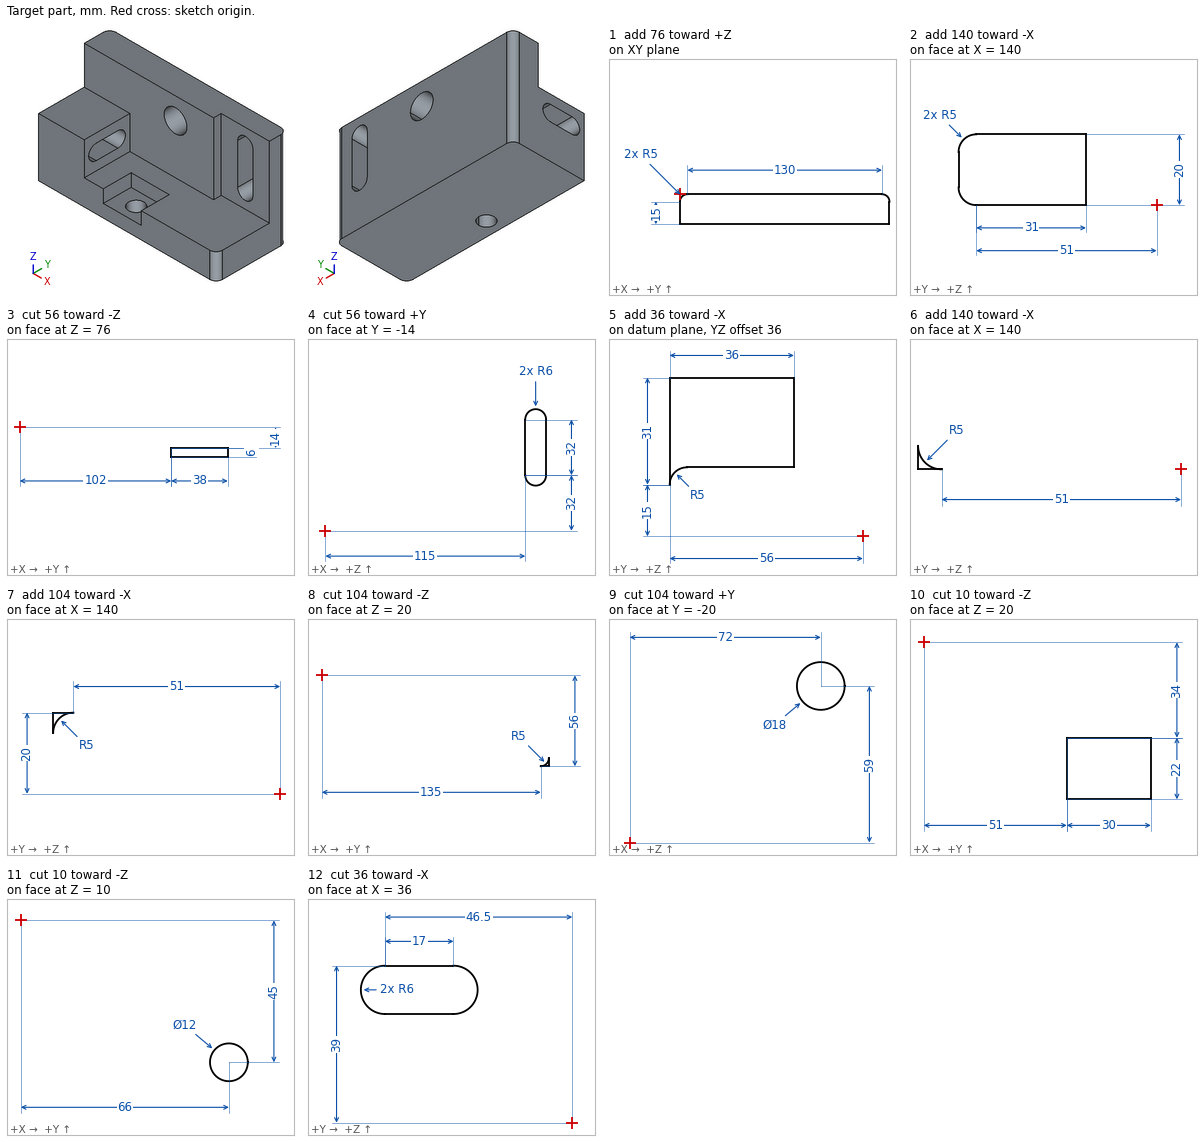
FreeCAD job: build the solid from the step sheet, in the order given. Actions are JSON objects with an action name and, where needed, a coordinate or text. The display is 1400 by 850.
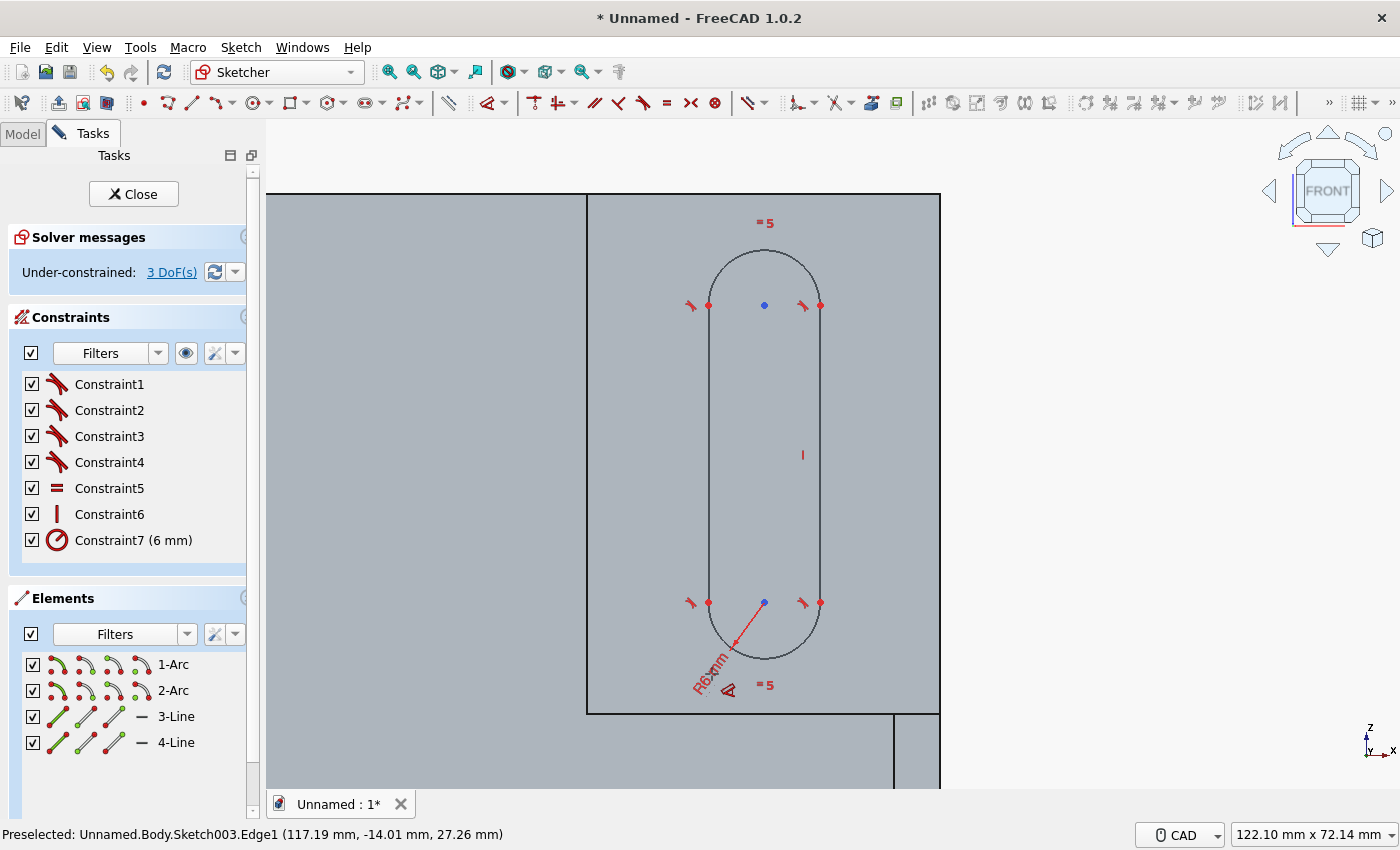
{"action": "left_click", "coordinate": [709, 514]}
{"action": "left_click", "coordinate": [675, 455]}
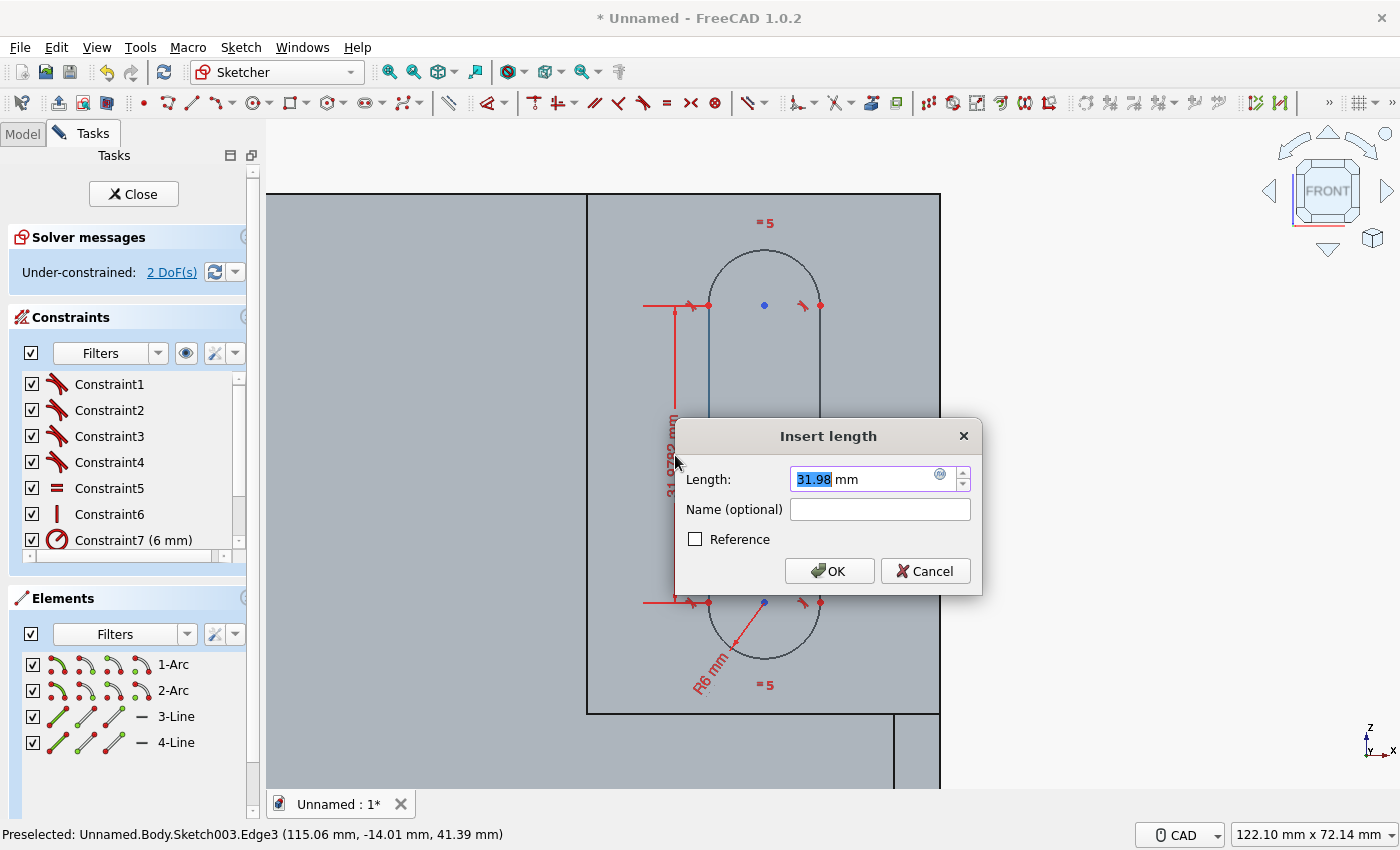
{"action": "type", "text": "32"}
{"action": "key", "text": "Return"}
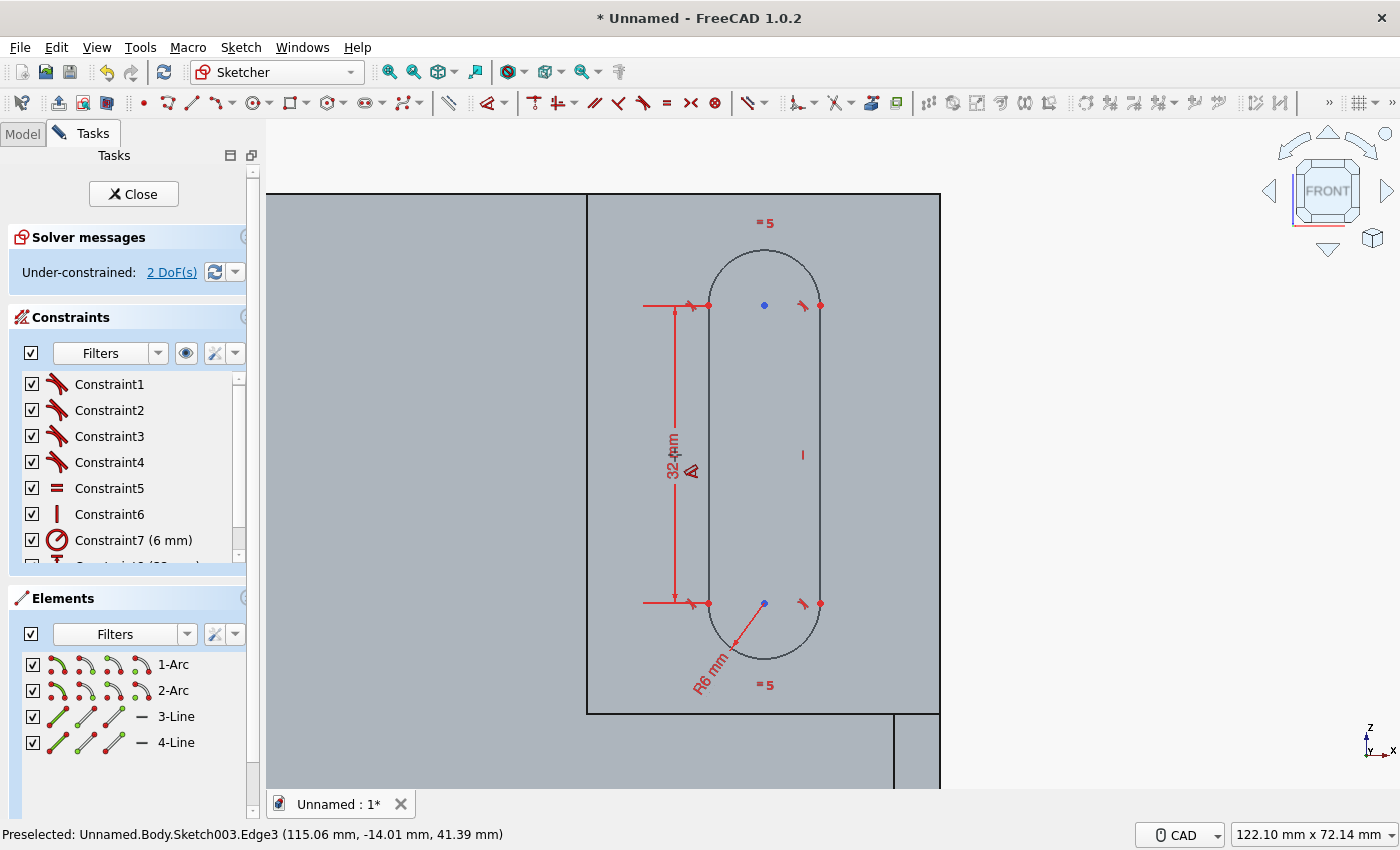
{"action": "left_click", "coordinate": [709, 603]}
{"action": "left_click", "coordinate": [743, 718]}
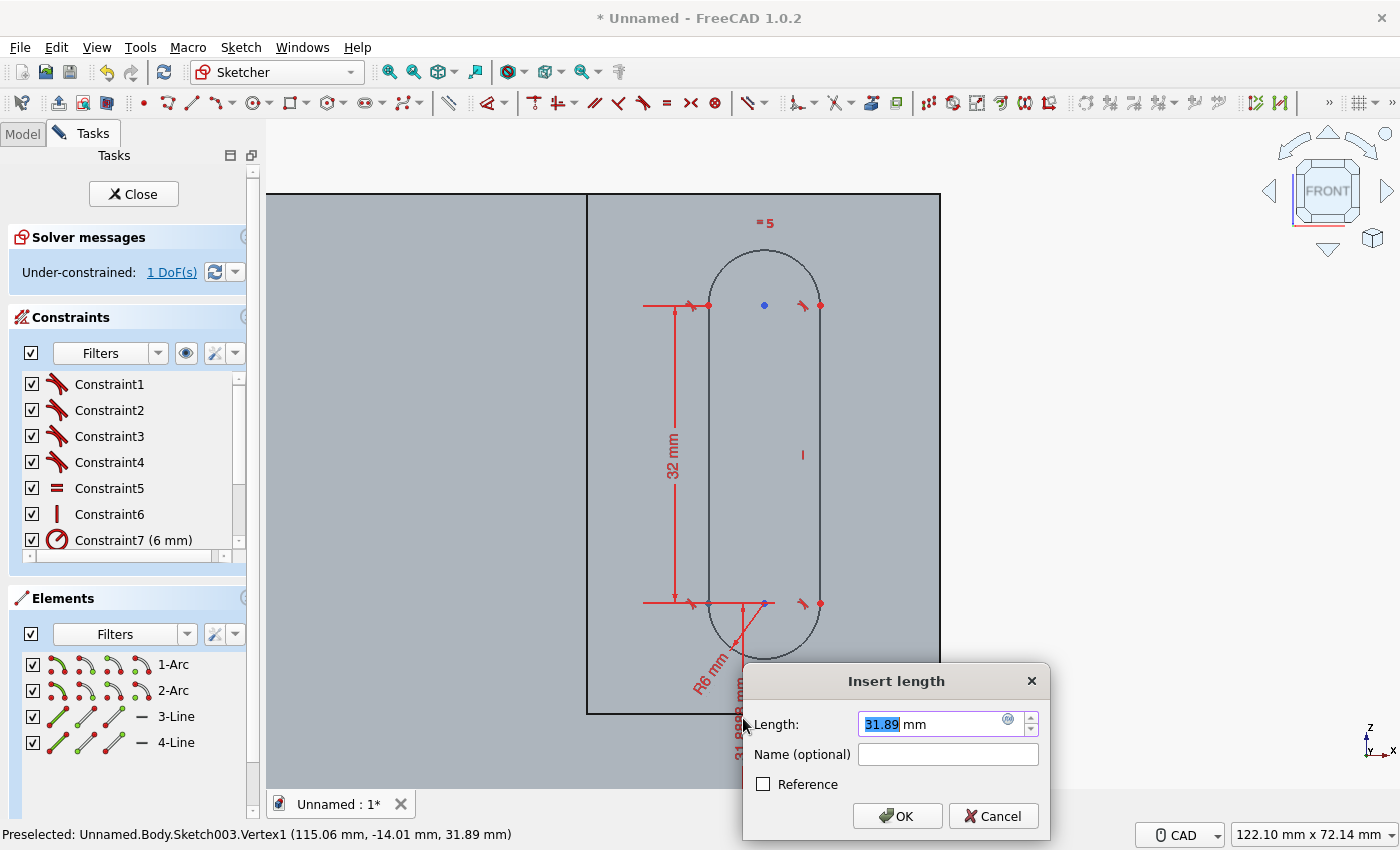
{"action": "type", "text": "32"}
{"action": "key", "text": "Return"}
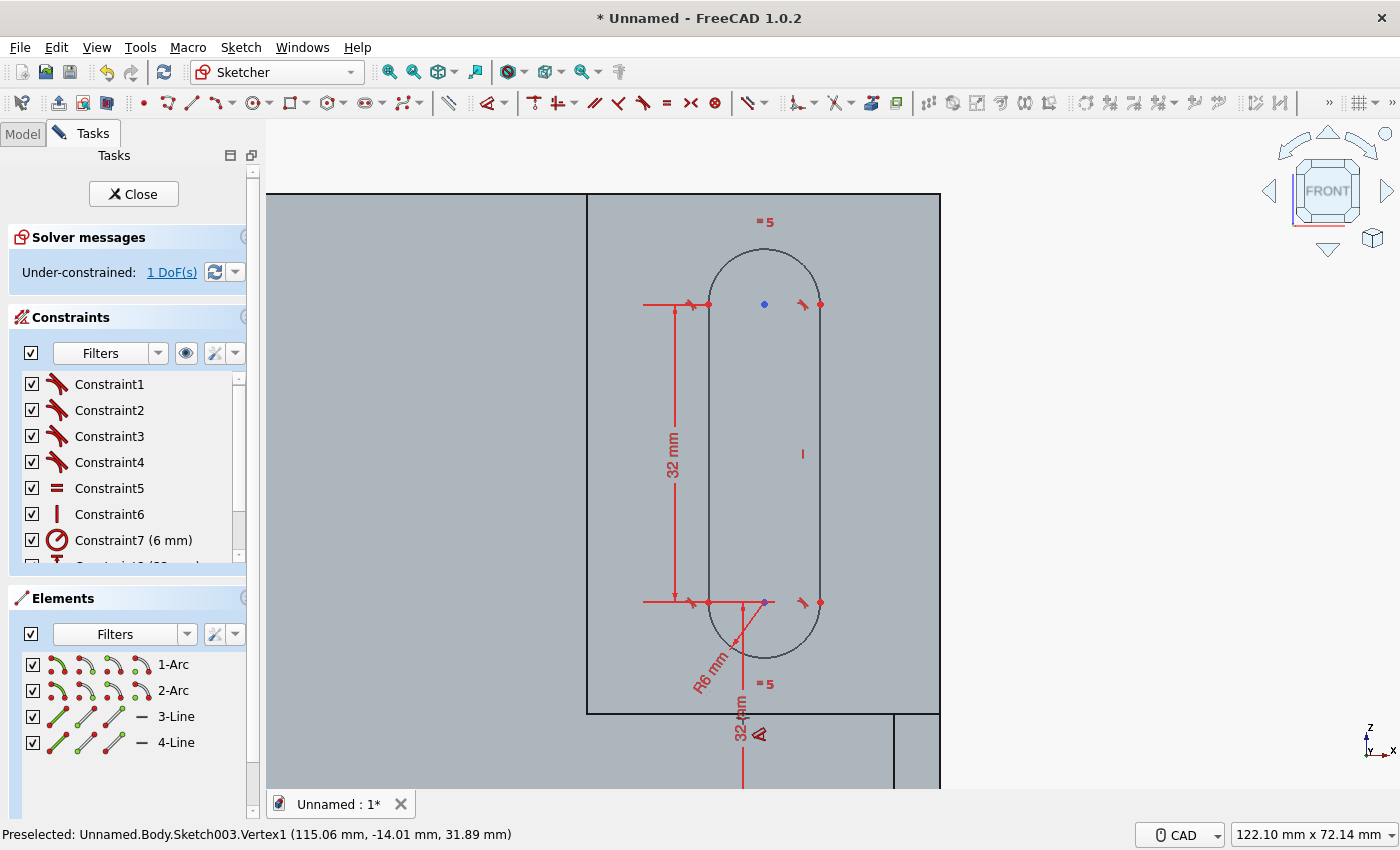
{"action": "left_click", "coordinate": [709, 602]}
{"action": "left_click", "coordinate": [501, 568]}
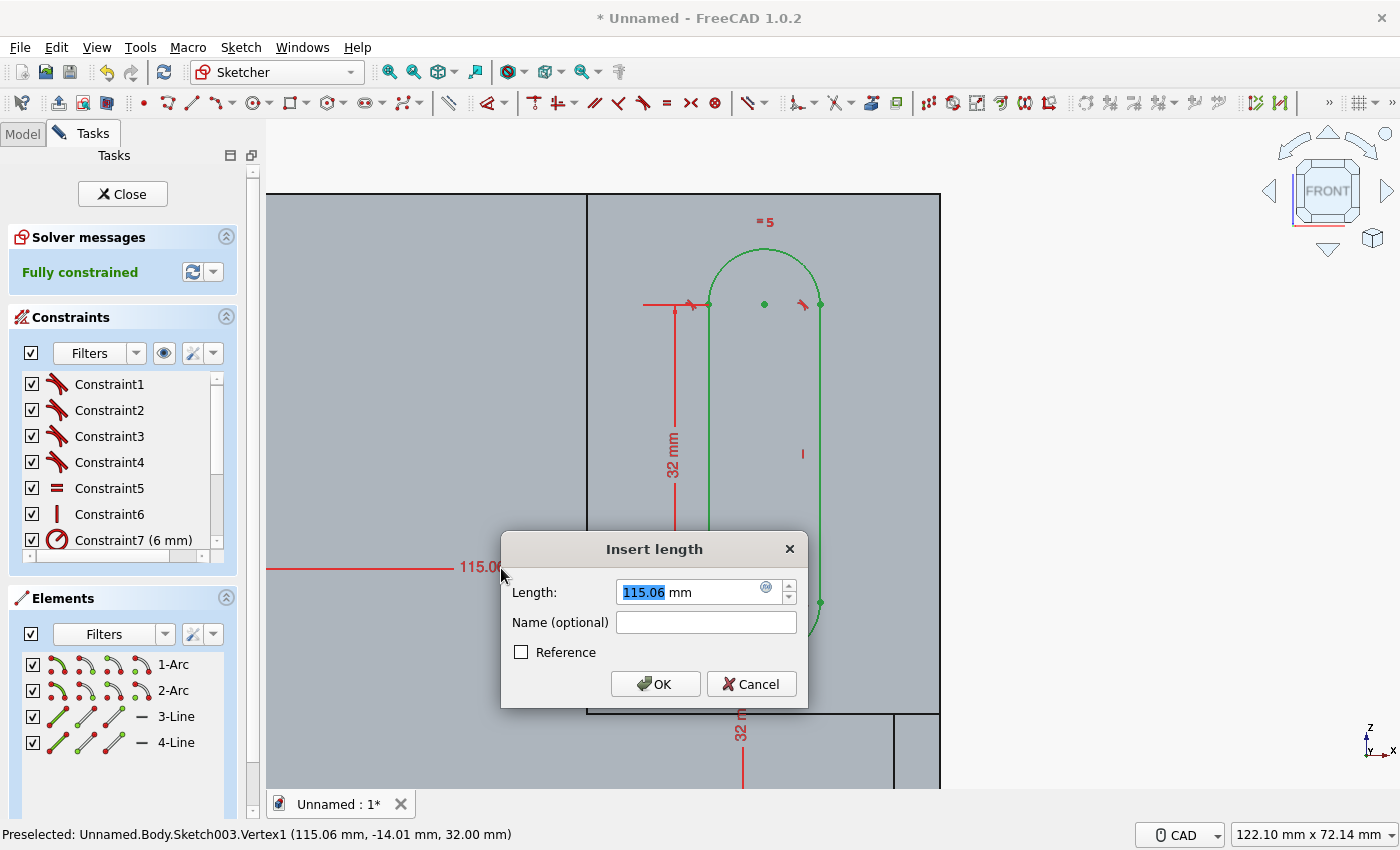
{"action": "type", "text": "115"}
{"action": "key", "text": "Return"}
{"action": "key", "text": "Escape"}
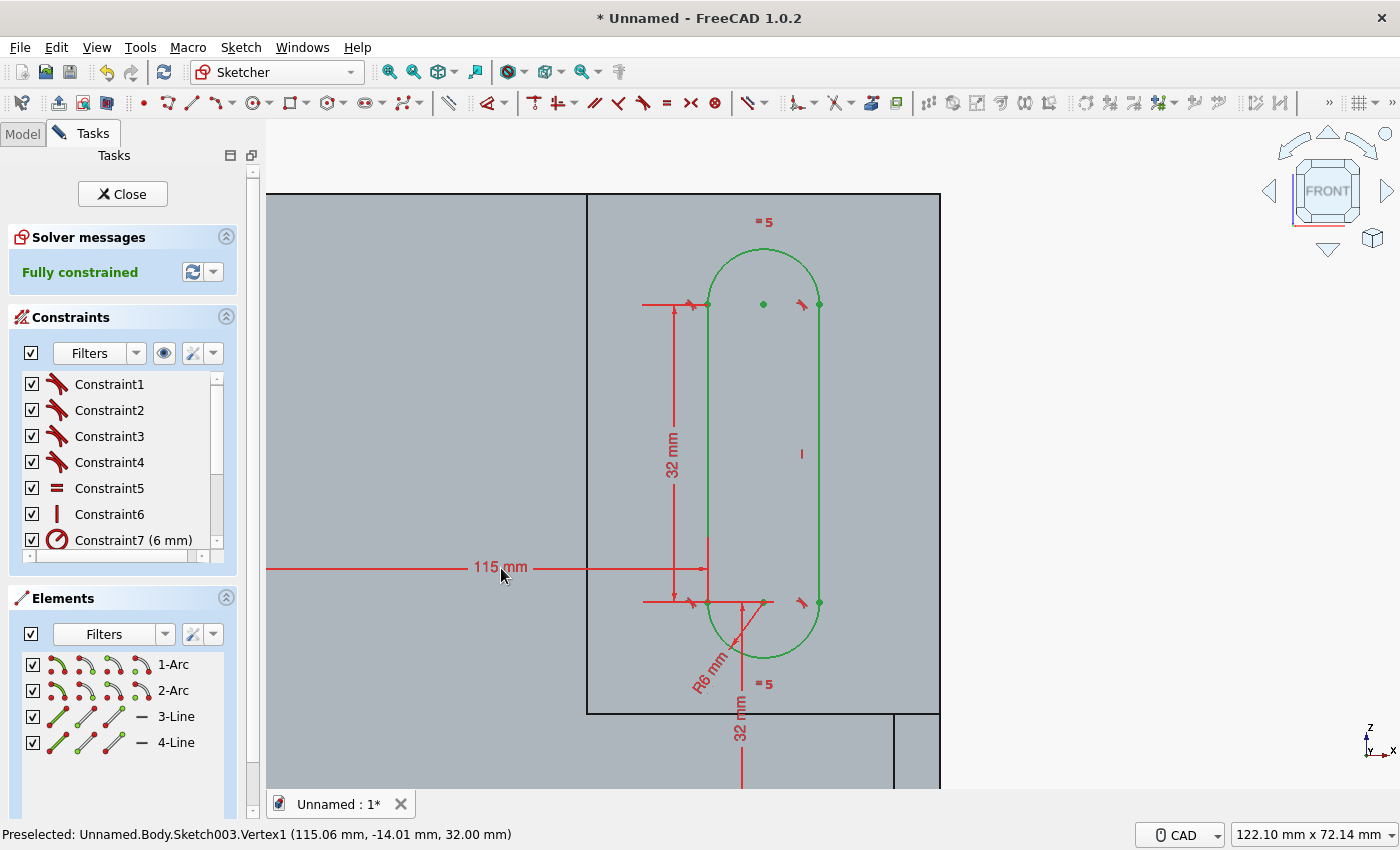
{"action": "left_click", "coordinate": [123, 194]}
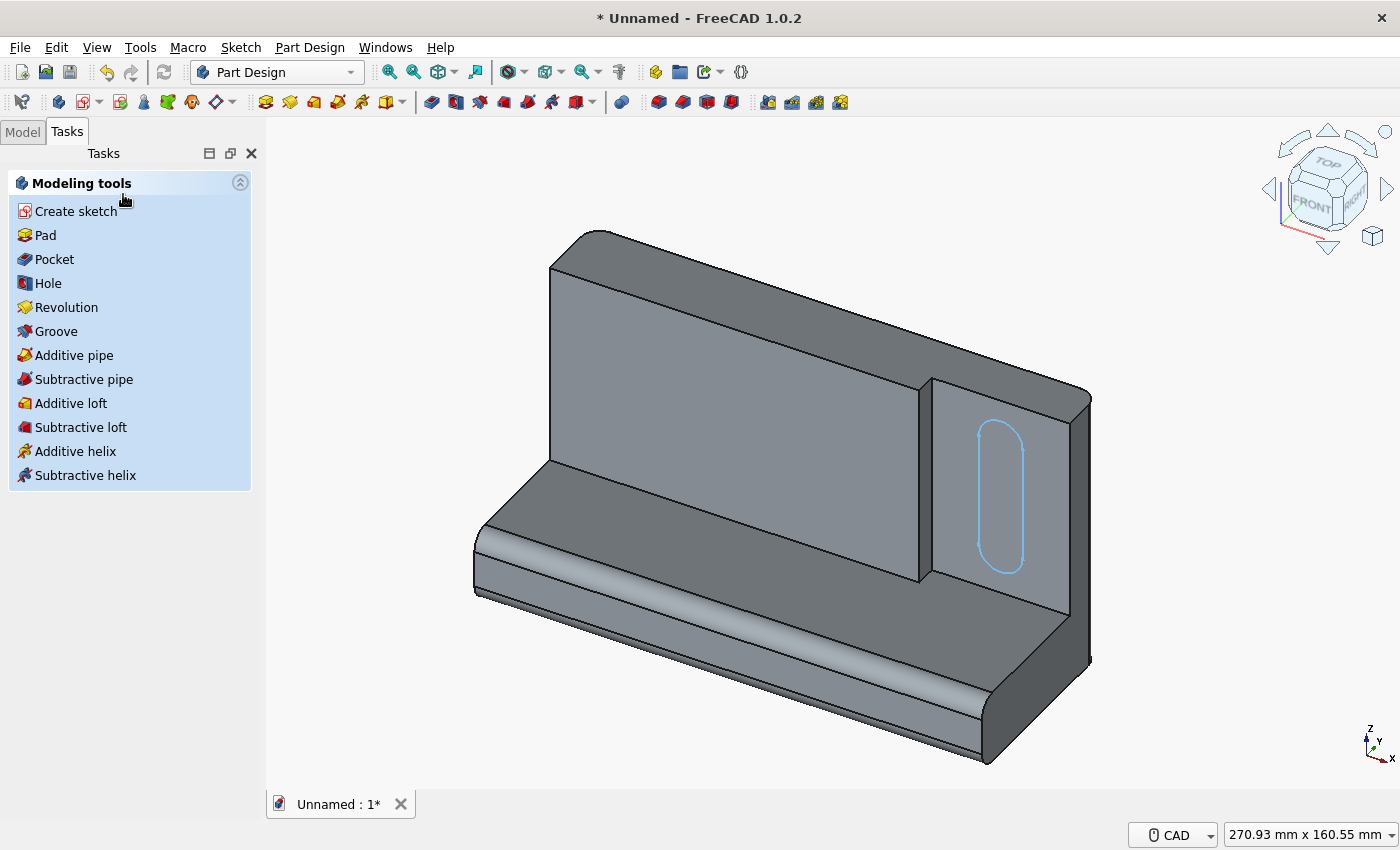
{"action": "left_click", "coordinate": [432, 102]}